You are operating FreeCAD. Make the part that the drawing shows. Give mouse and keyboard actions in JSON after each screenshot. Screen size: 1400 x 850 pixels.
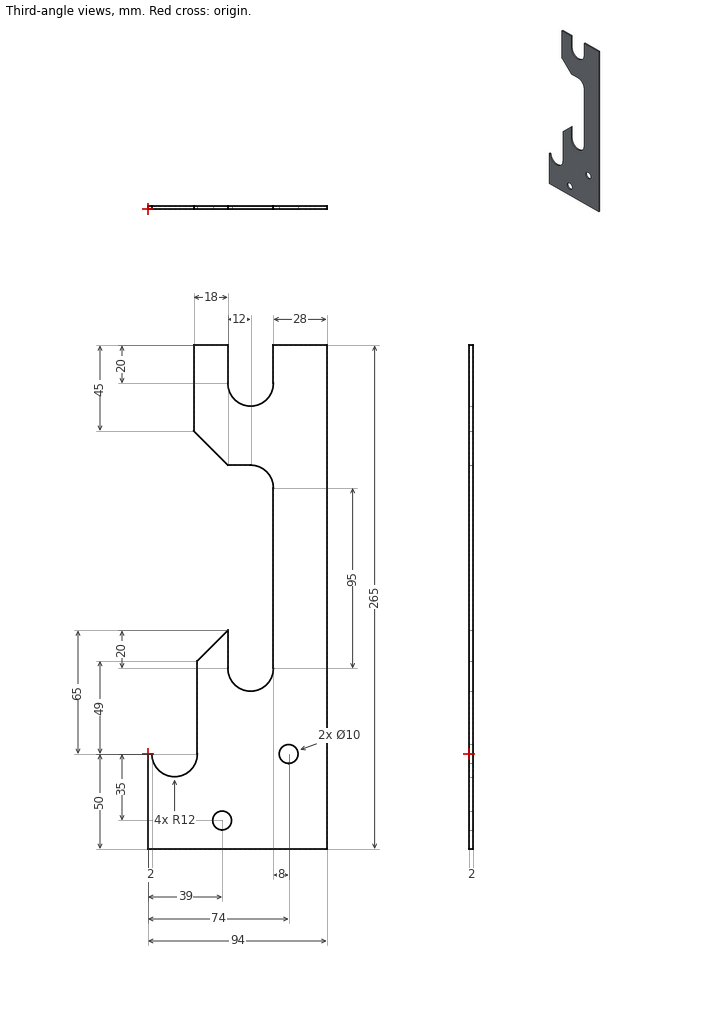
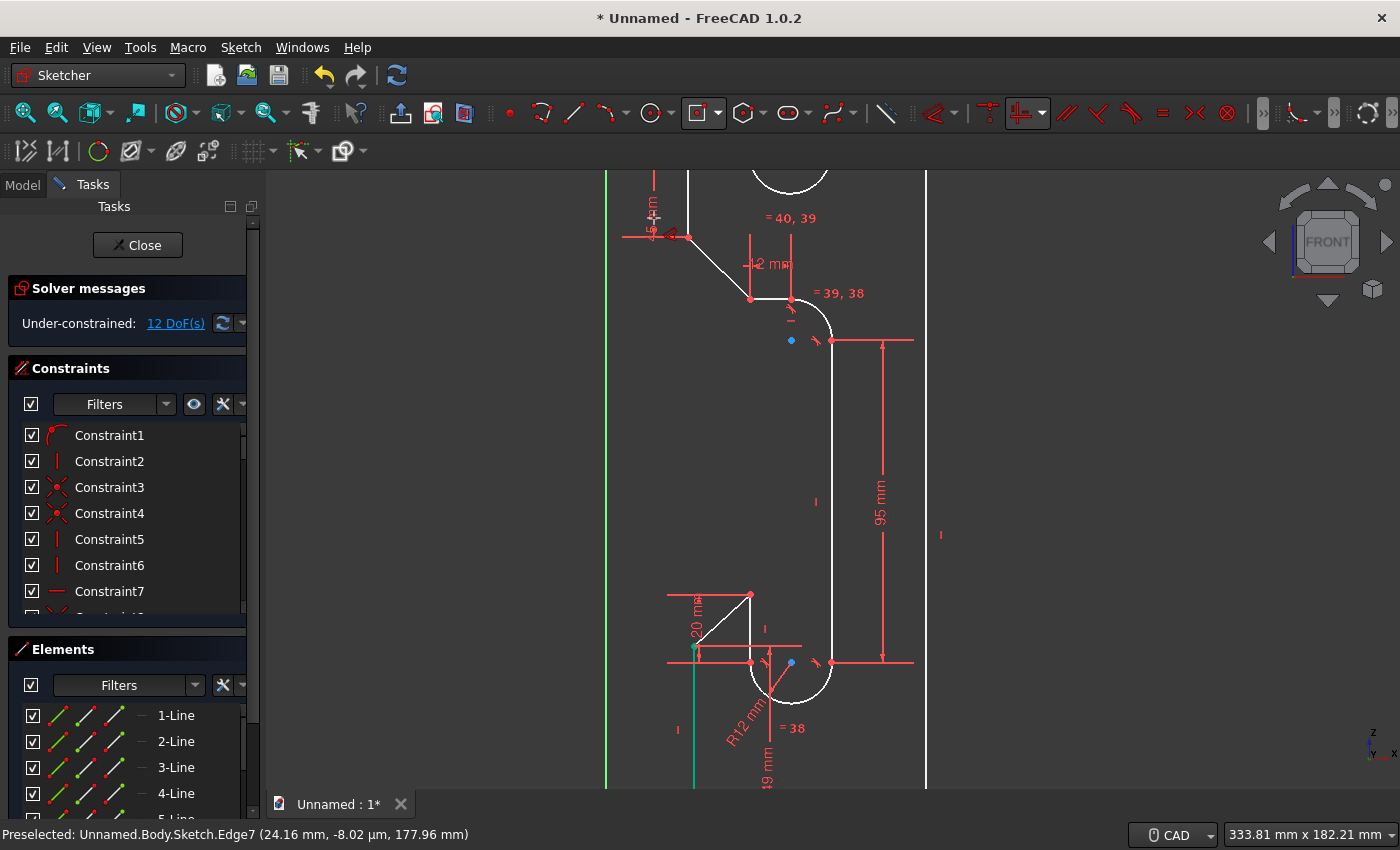
{"action": "scroll", "coordinate": [763, 436], "scroll_direction": "down", "scroll_amount": 4}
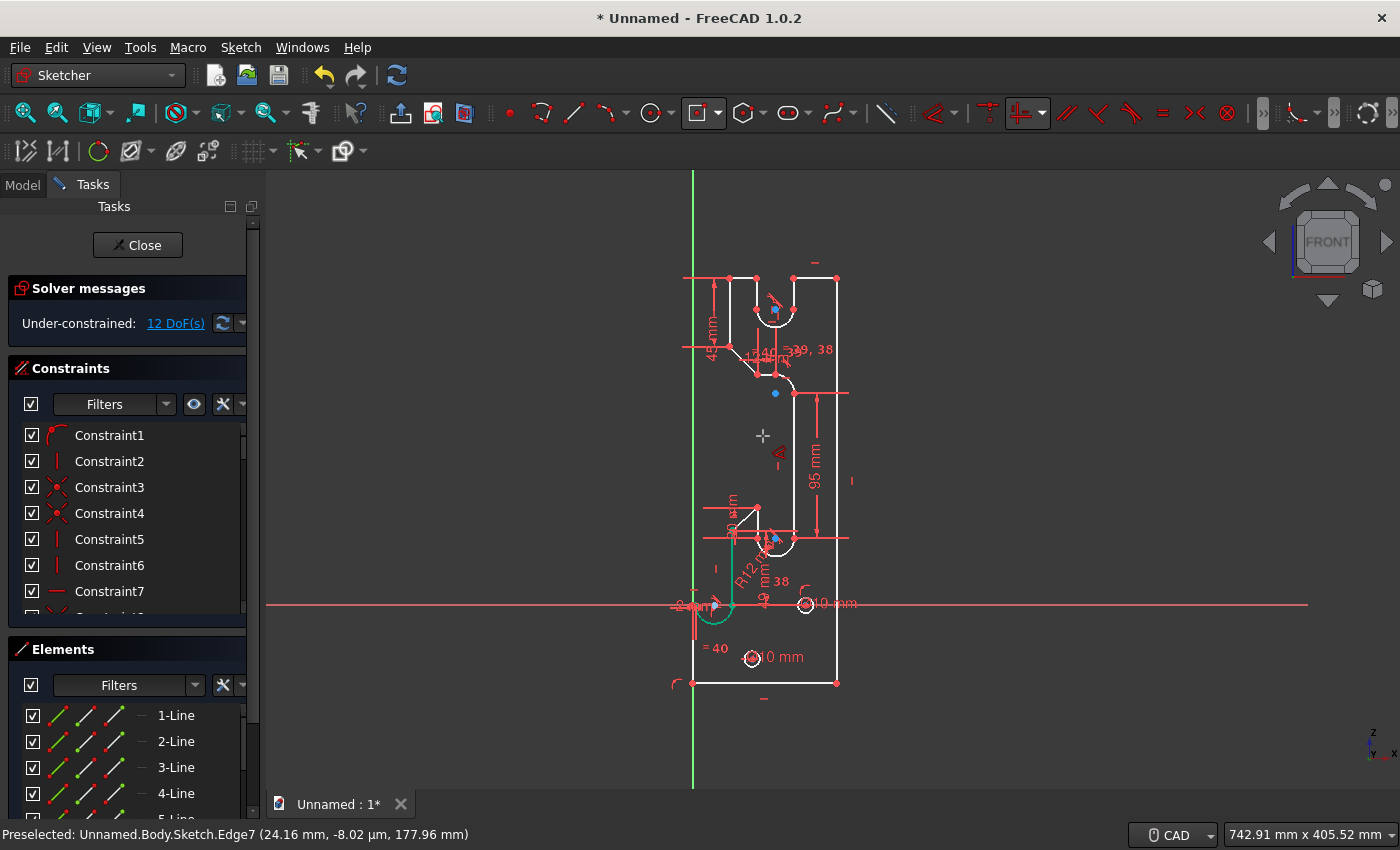
{"action": "scroll", "coordinate": [738, 278], "scroll_direction": "up", "scroll_amount": 3}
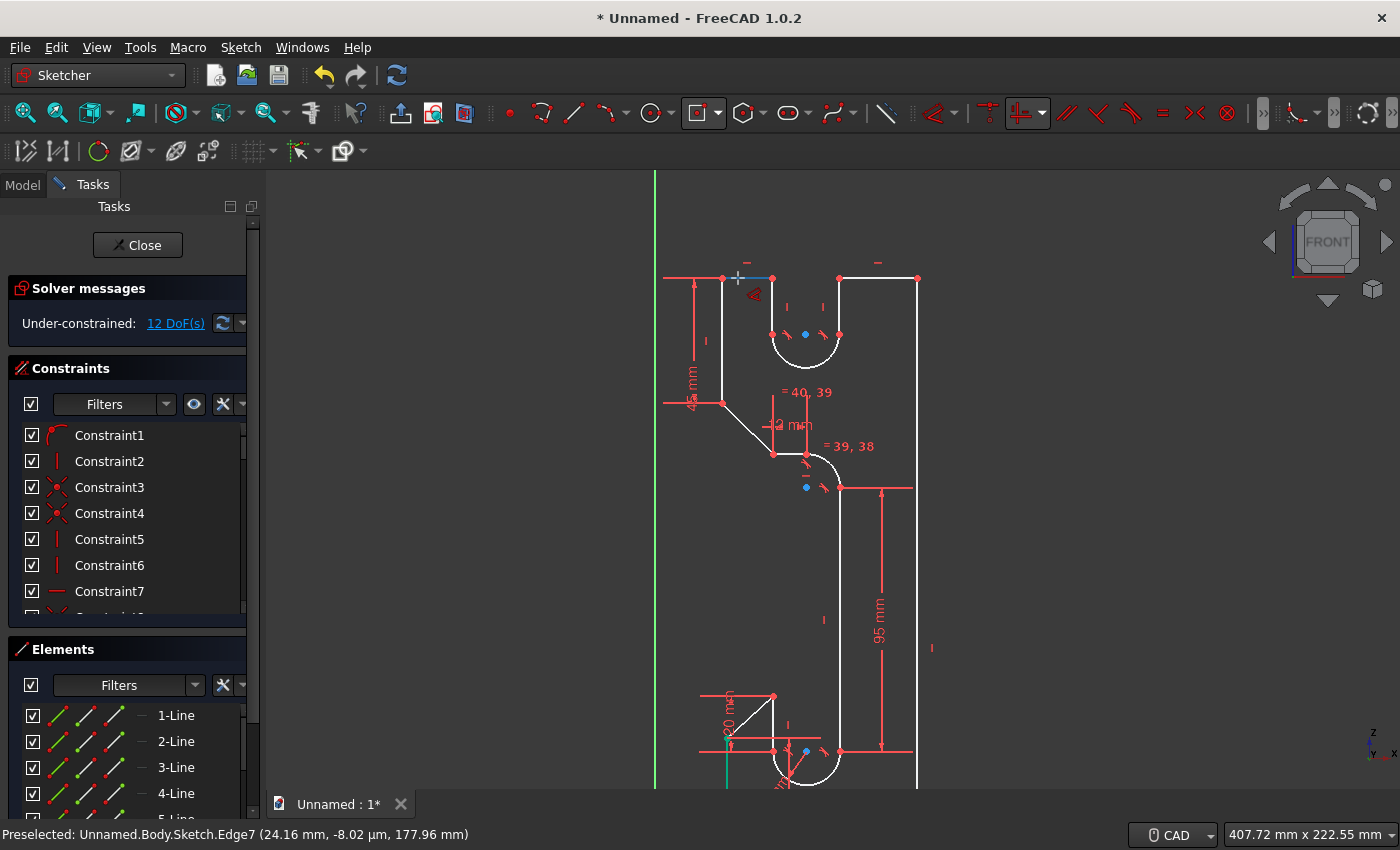
{"action": "left_click", "coordinate": [737, 278]}
{"action": "left_click", "coordinate": [747, 244]}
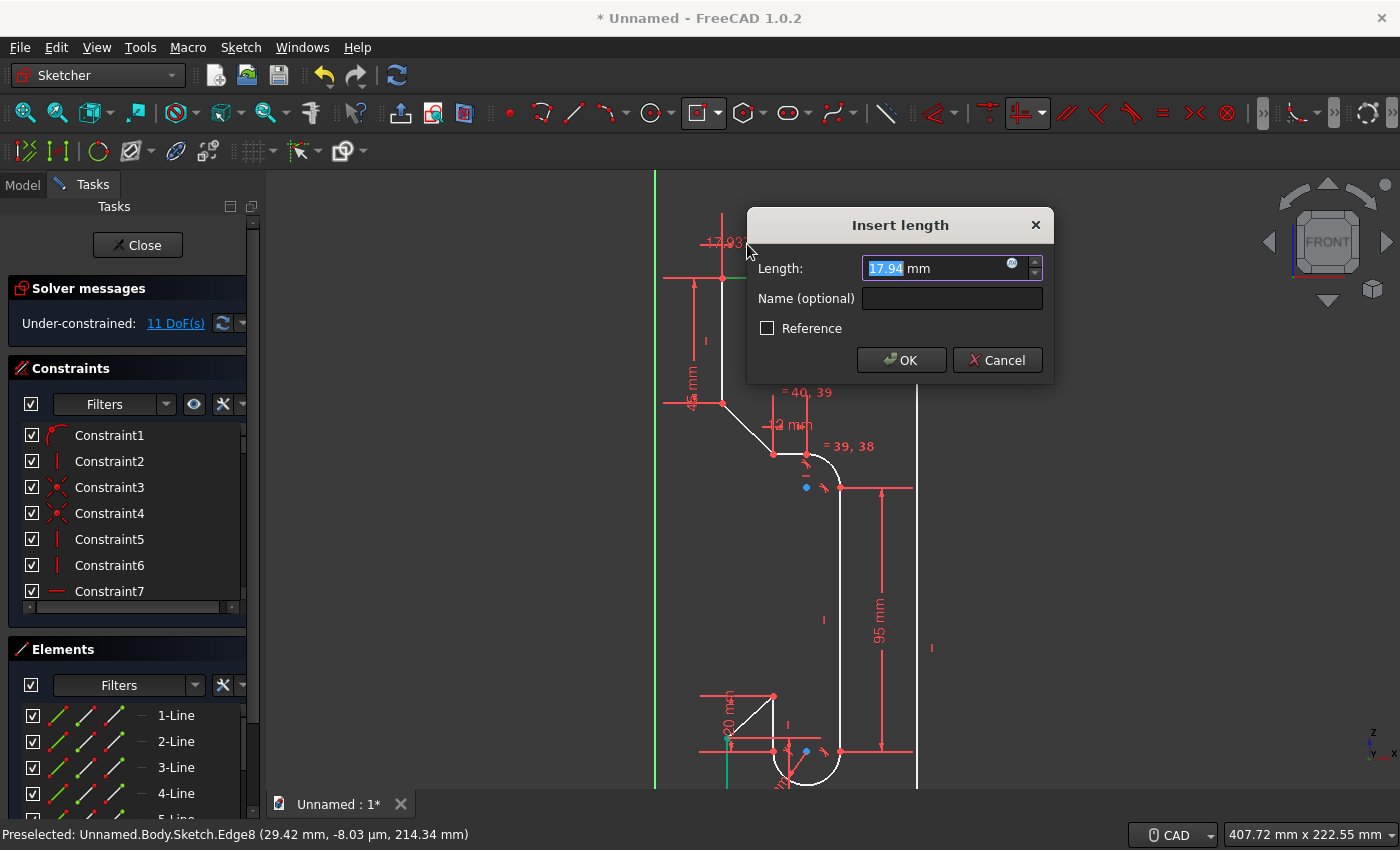
{"action": "type", "text": "18"}
{"action": "key", "text": "Return"}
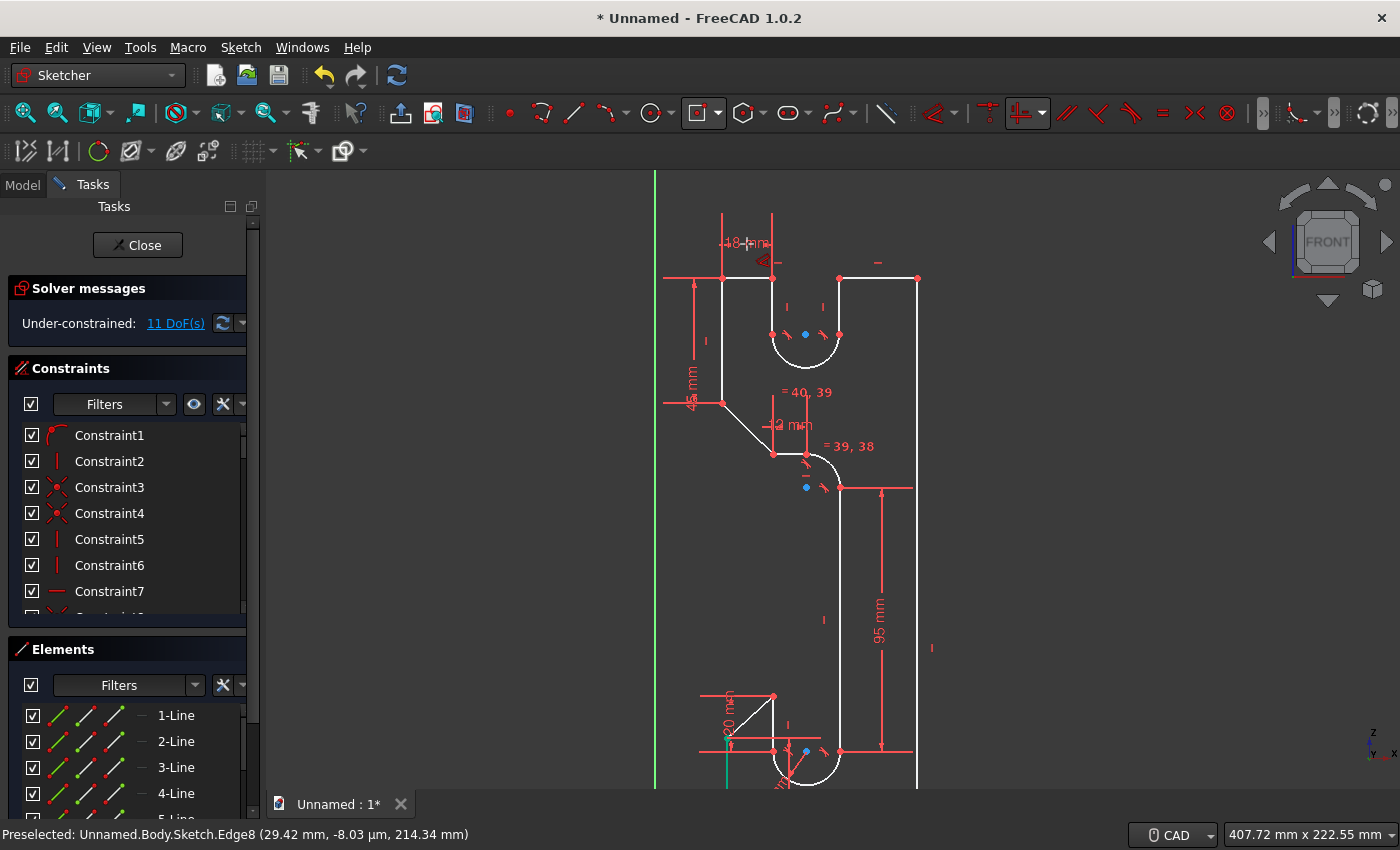
{"action": "left_click", "coordinate": [772, 295]}
{"action": "left_click", "coordinate": [738, 306]}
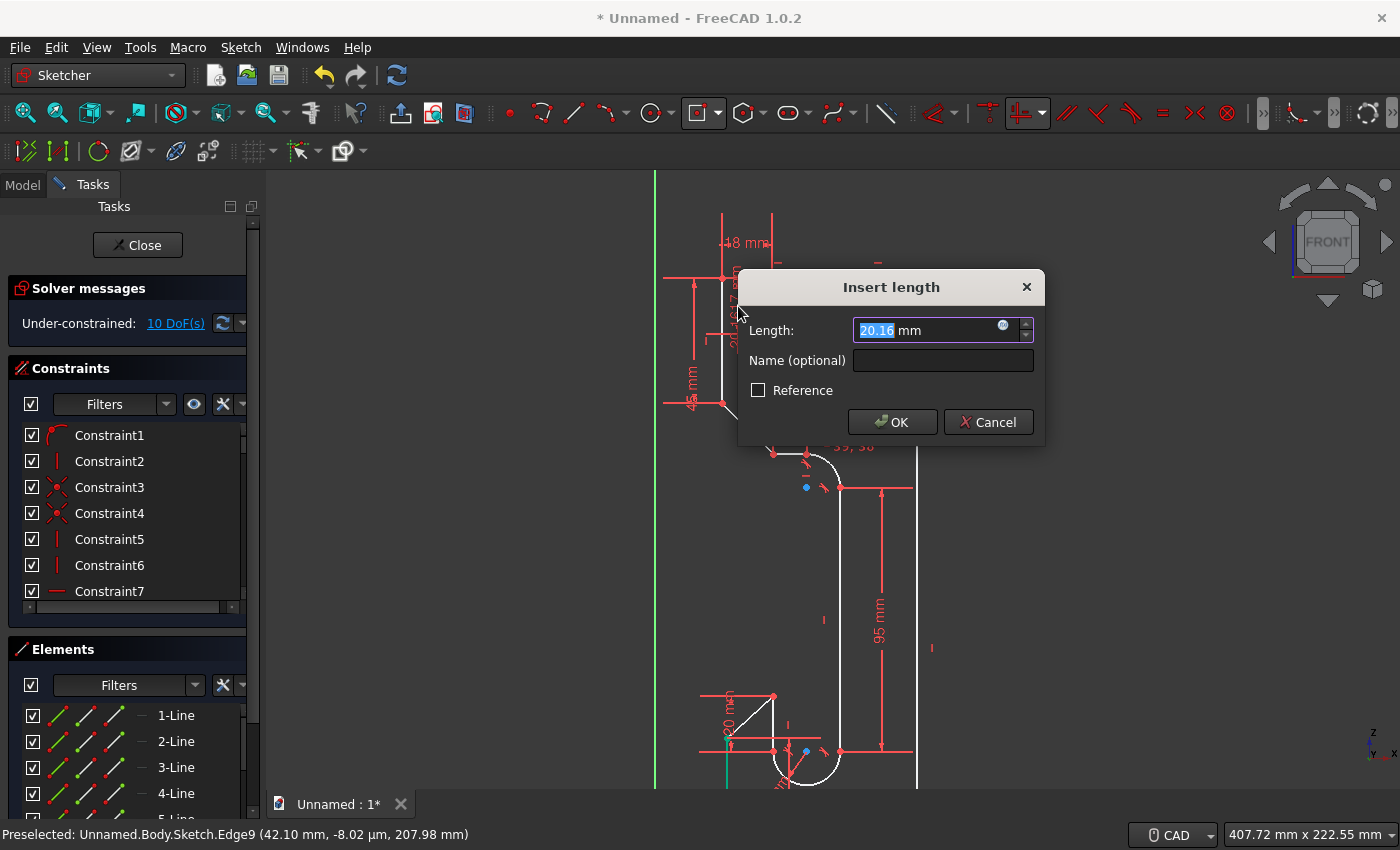
{"action": "type", "text": "20"}
{"action": "key", "text": "Return"}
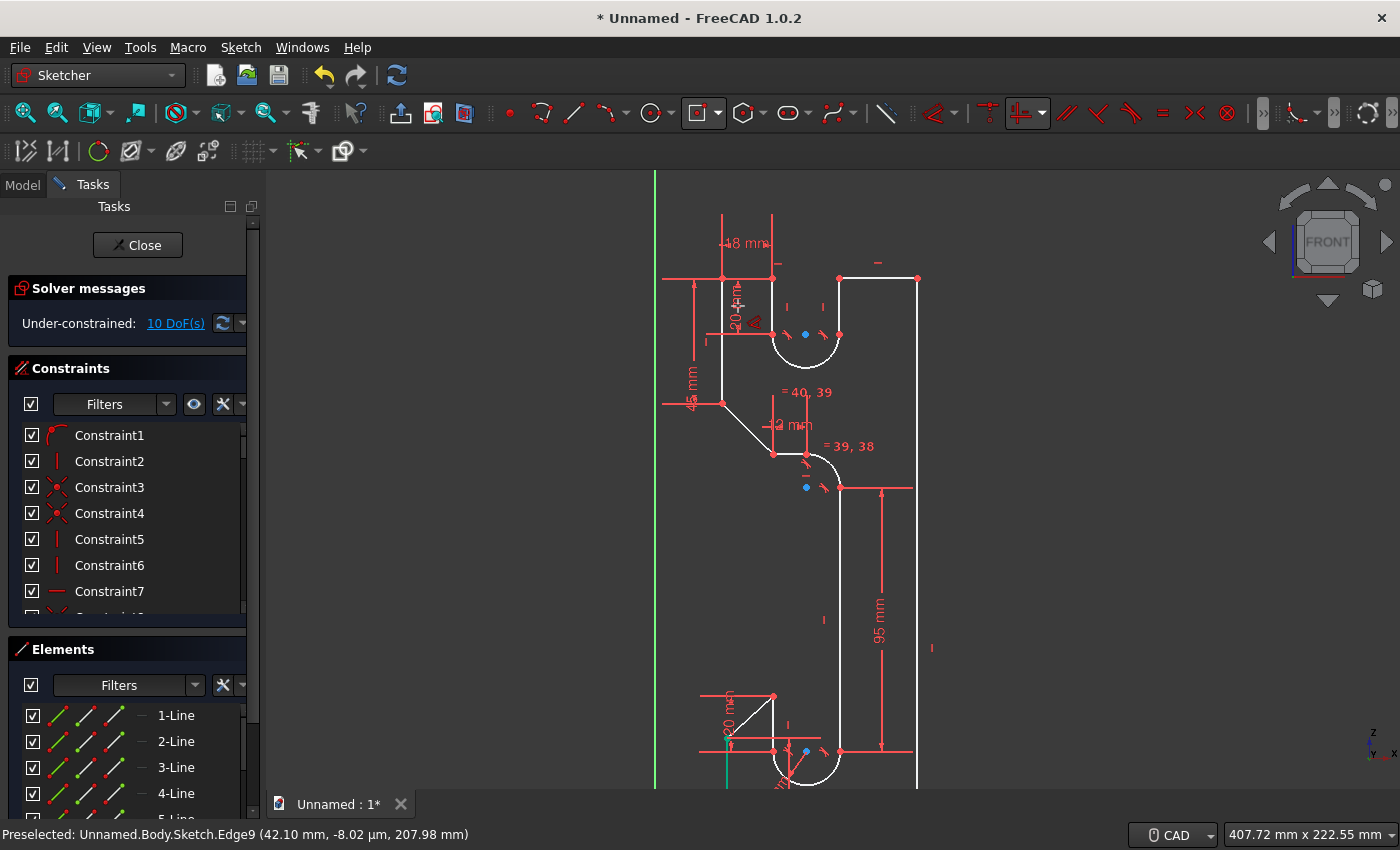
{"action": "left_click", "coordinate": [839, 318]}
{"action": "left_click", "coordinate": [873, 306]}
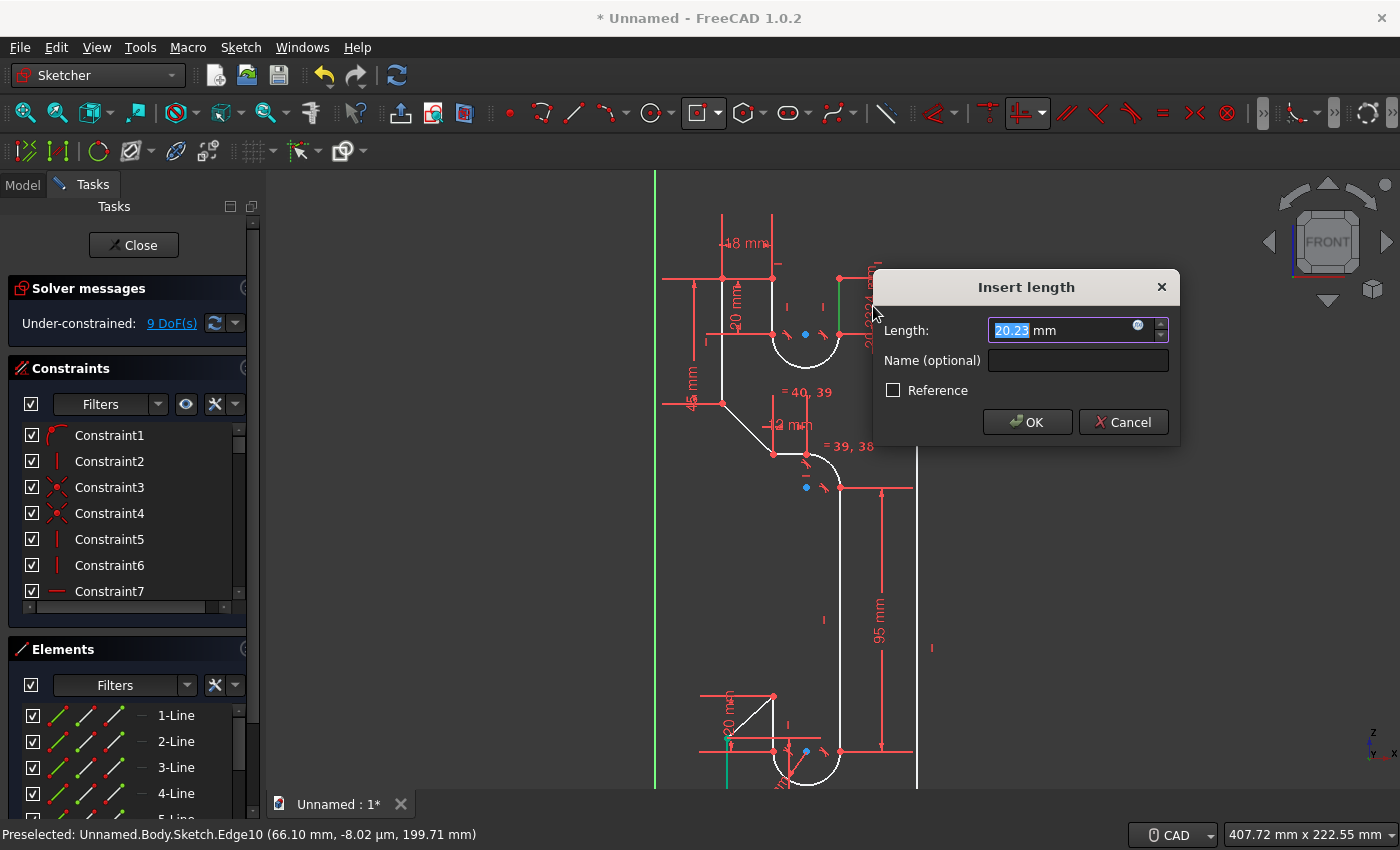
{"action": "type", "text": "20"}
{"action": "key", "text": "Return"}